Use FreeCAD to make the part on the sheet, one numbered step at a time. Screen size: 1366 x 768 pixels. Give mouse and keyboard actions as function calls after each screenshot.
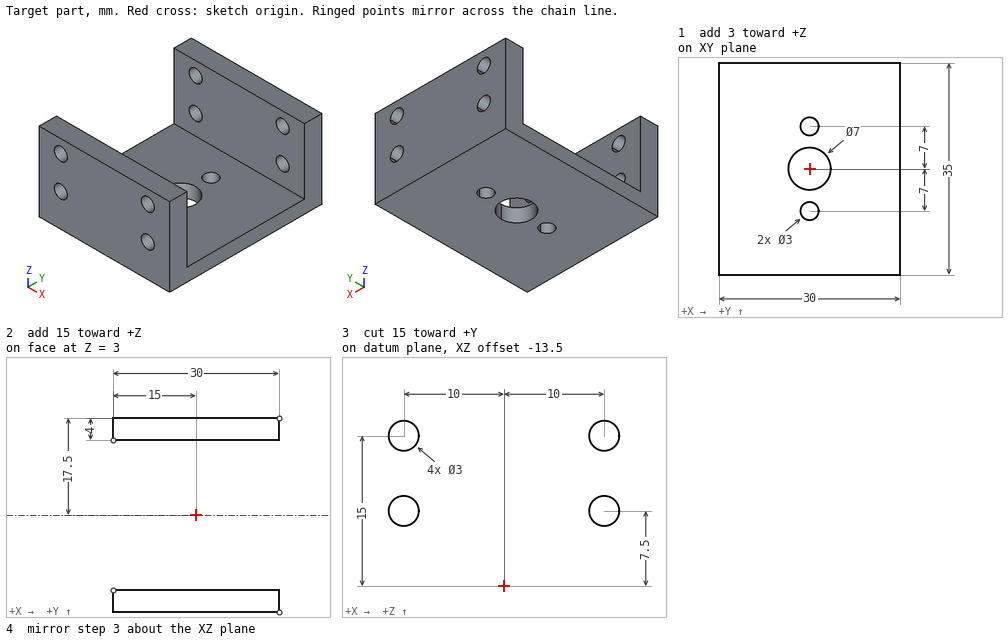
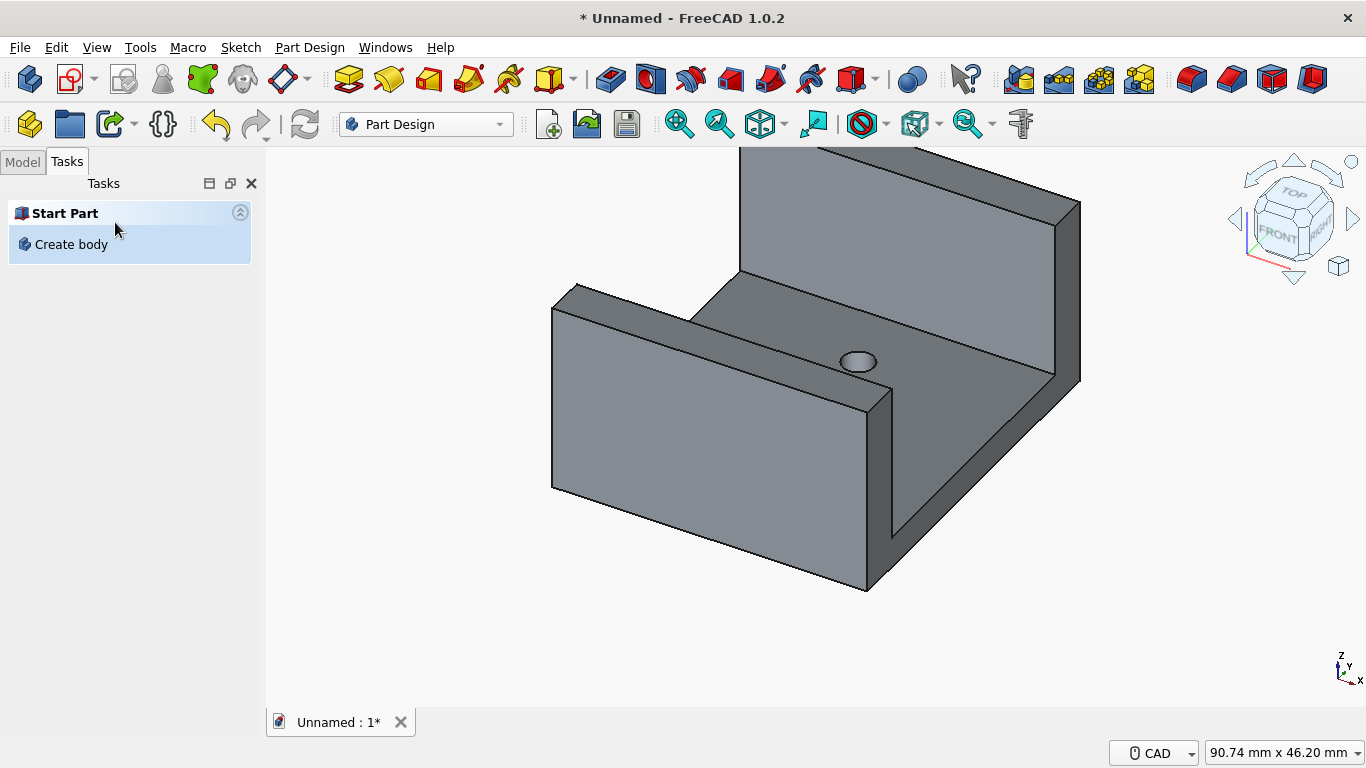
click(680, 124)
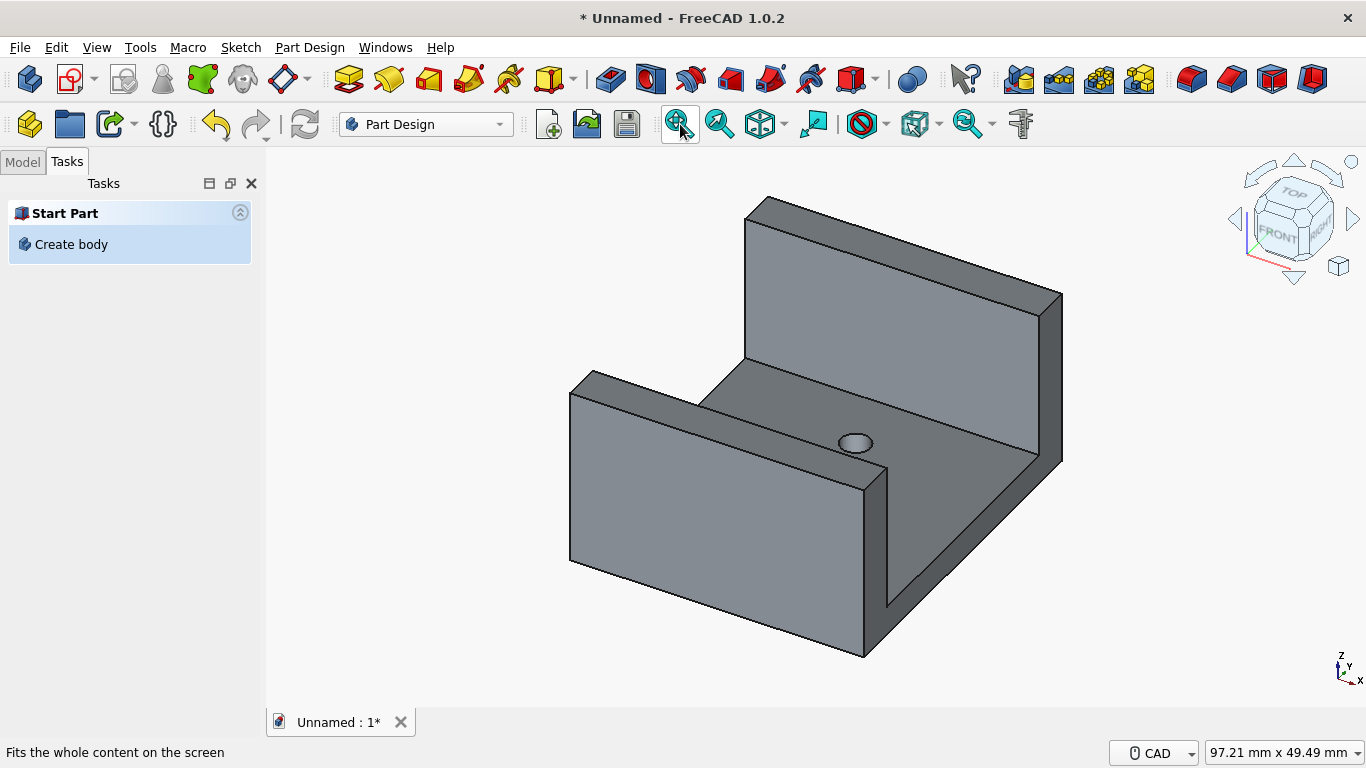
click(23, 161)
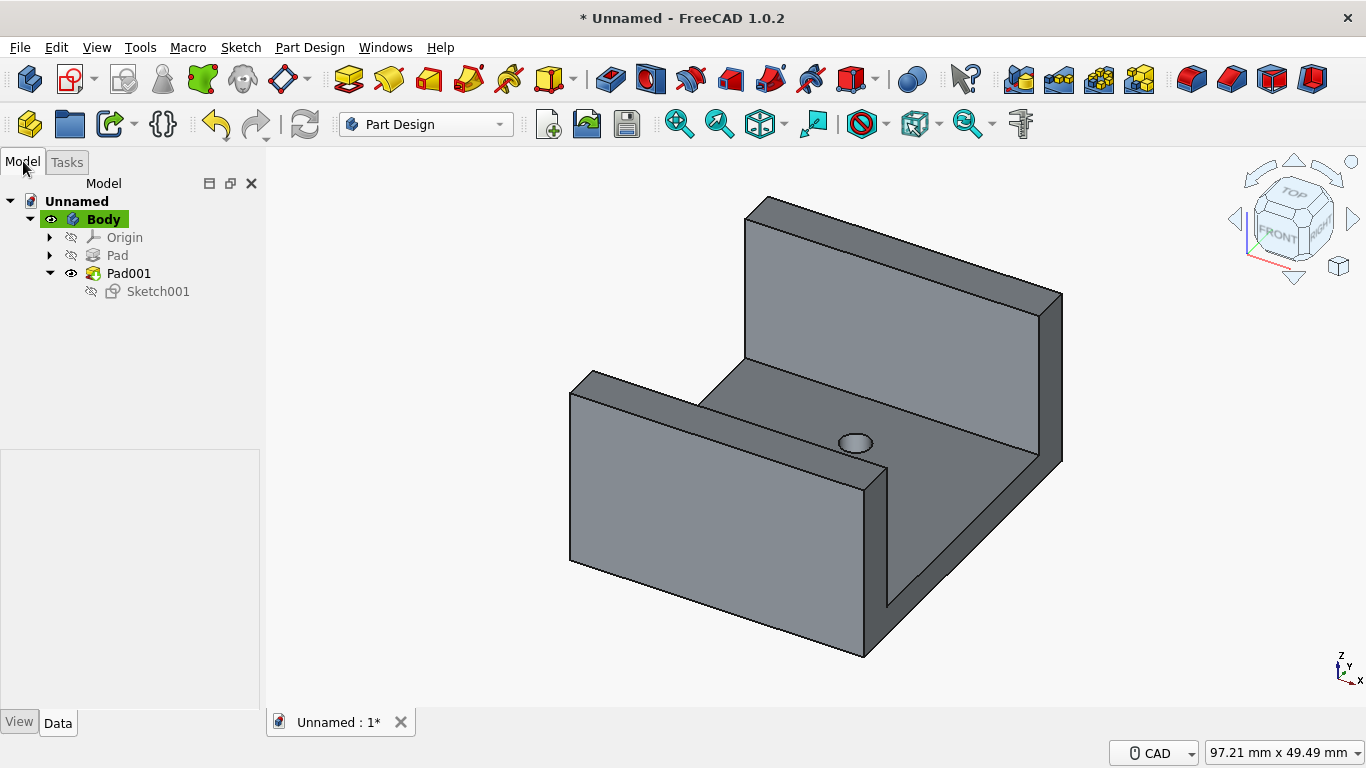
click(50, 237)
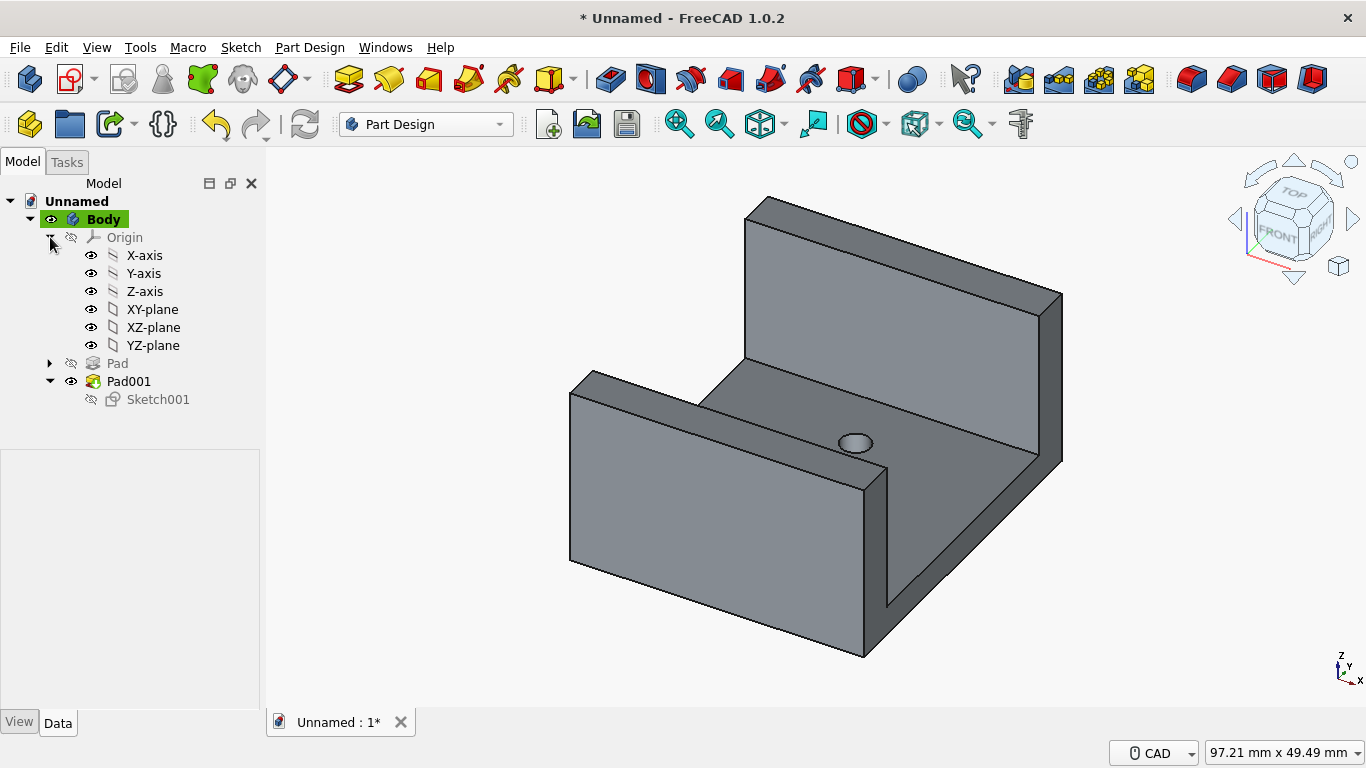
click(136, 327)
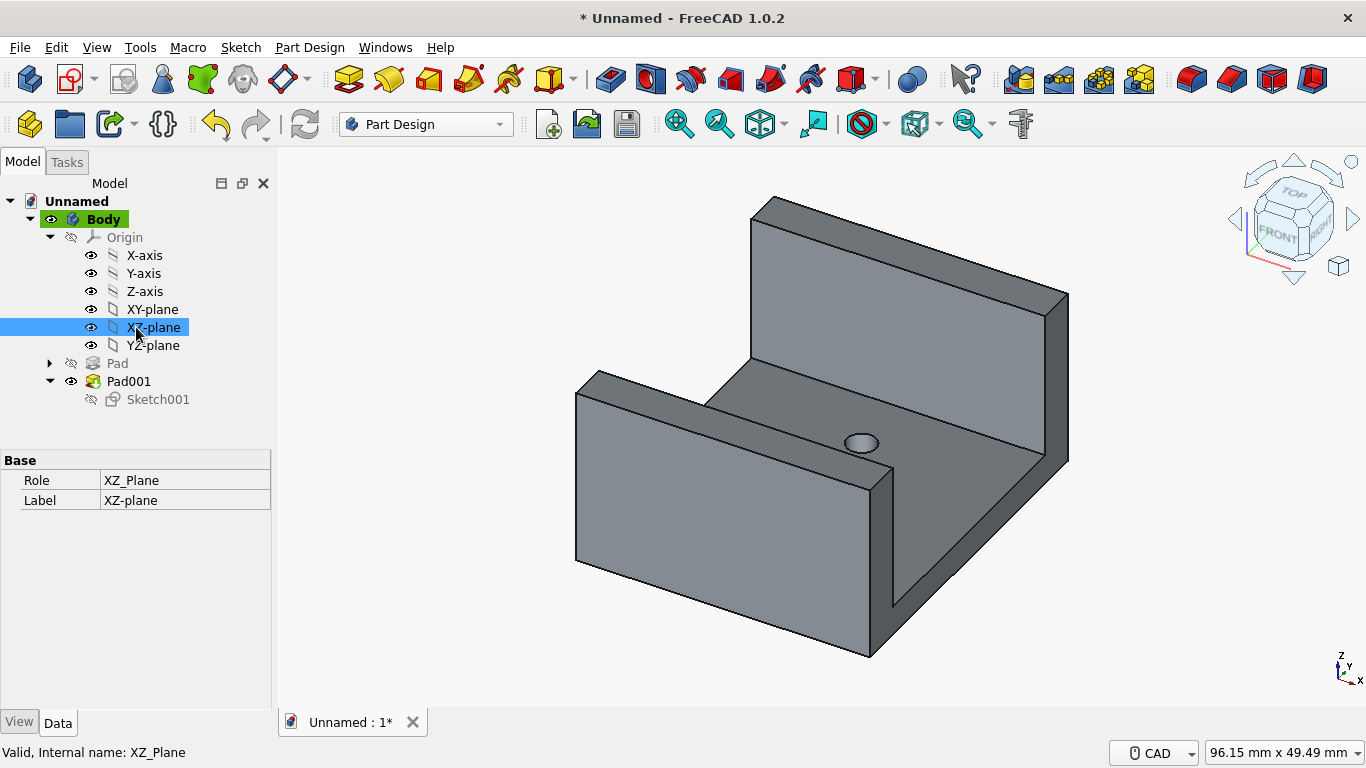
click(284, 80)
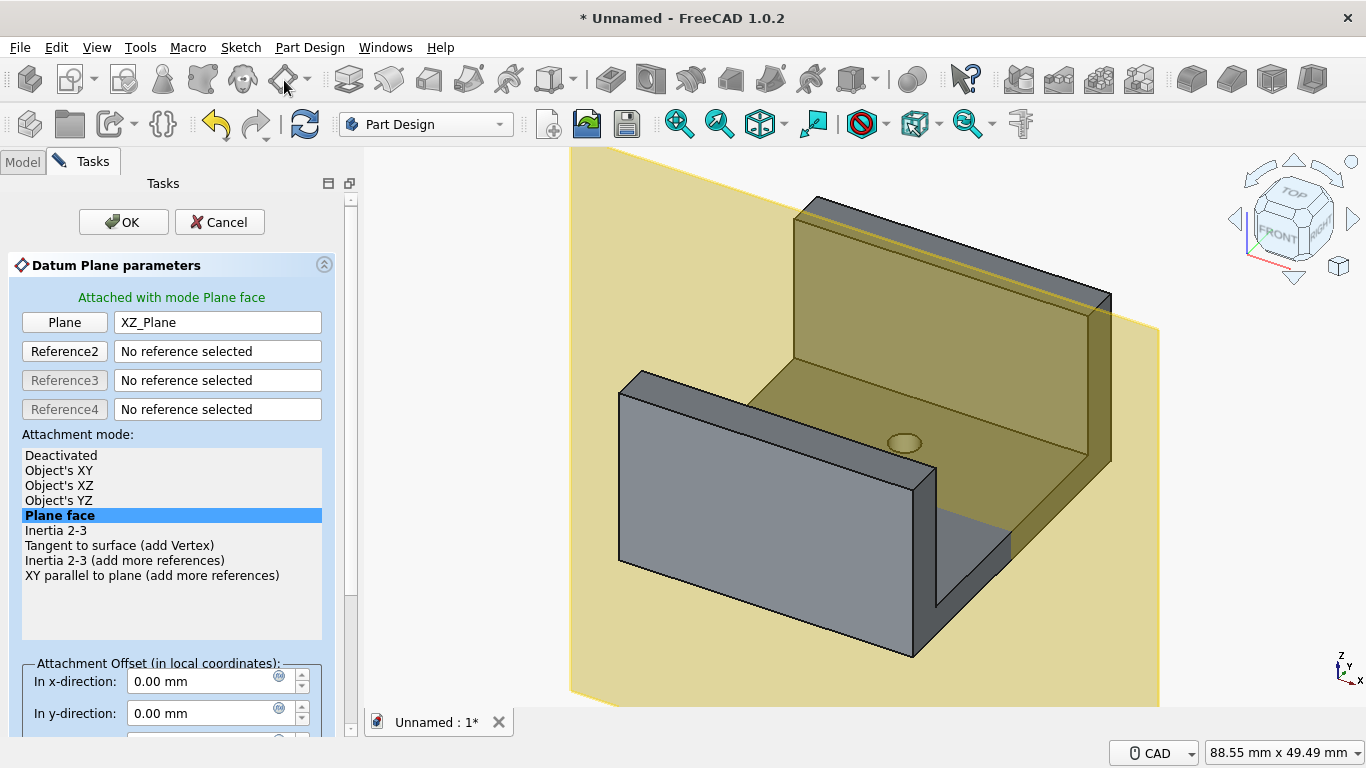
scroll(351, 464, down, 2)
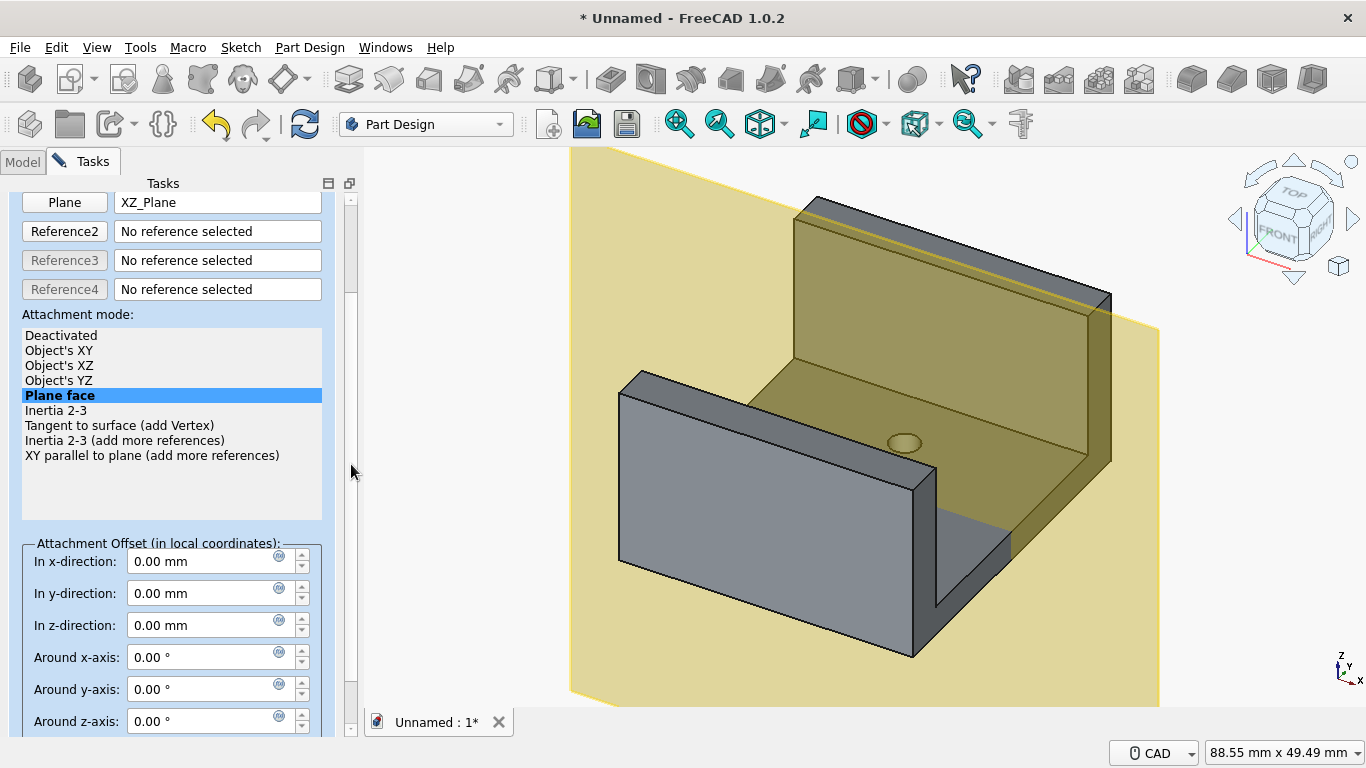
triple_click(210, 625)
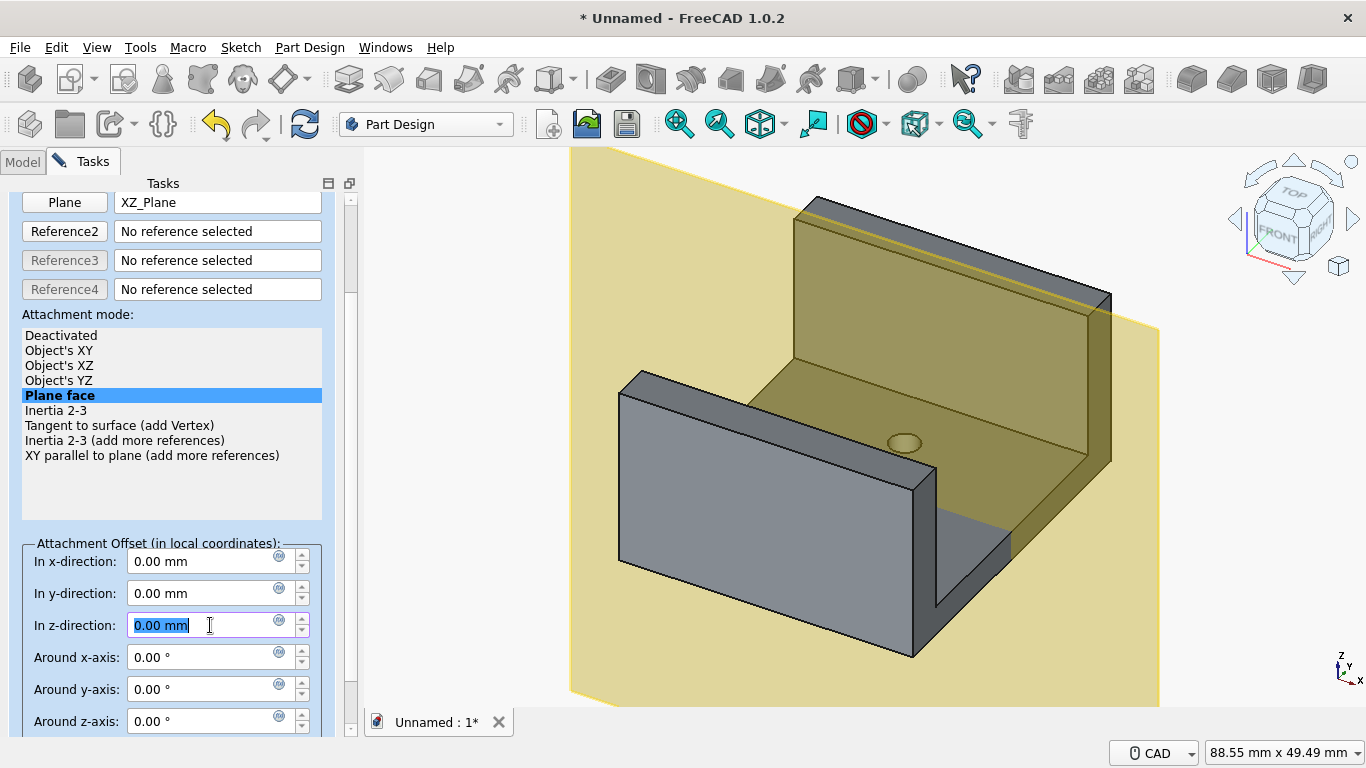
text(-13.5)
key(Tab)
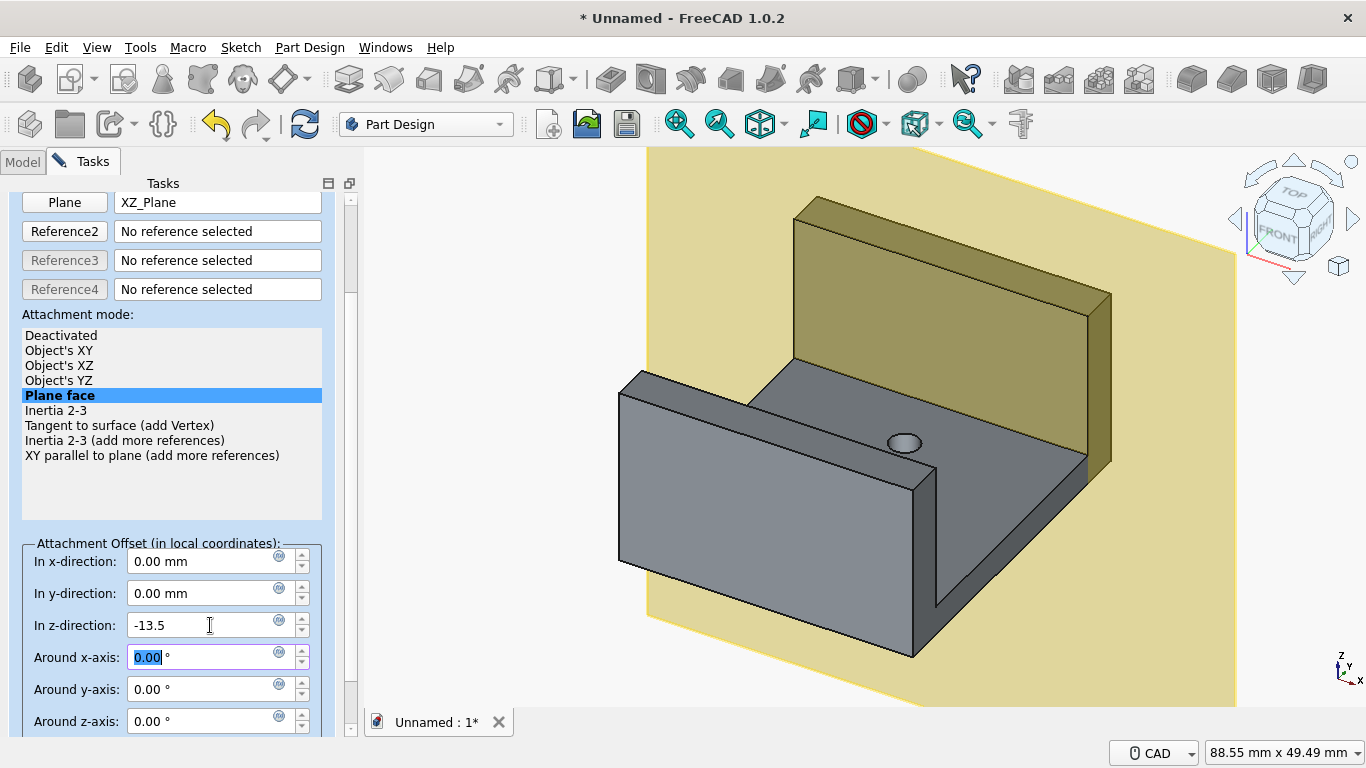
scroll(351, 464, up, 3)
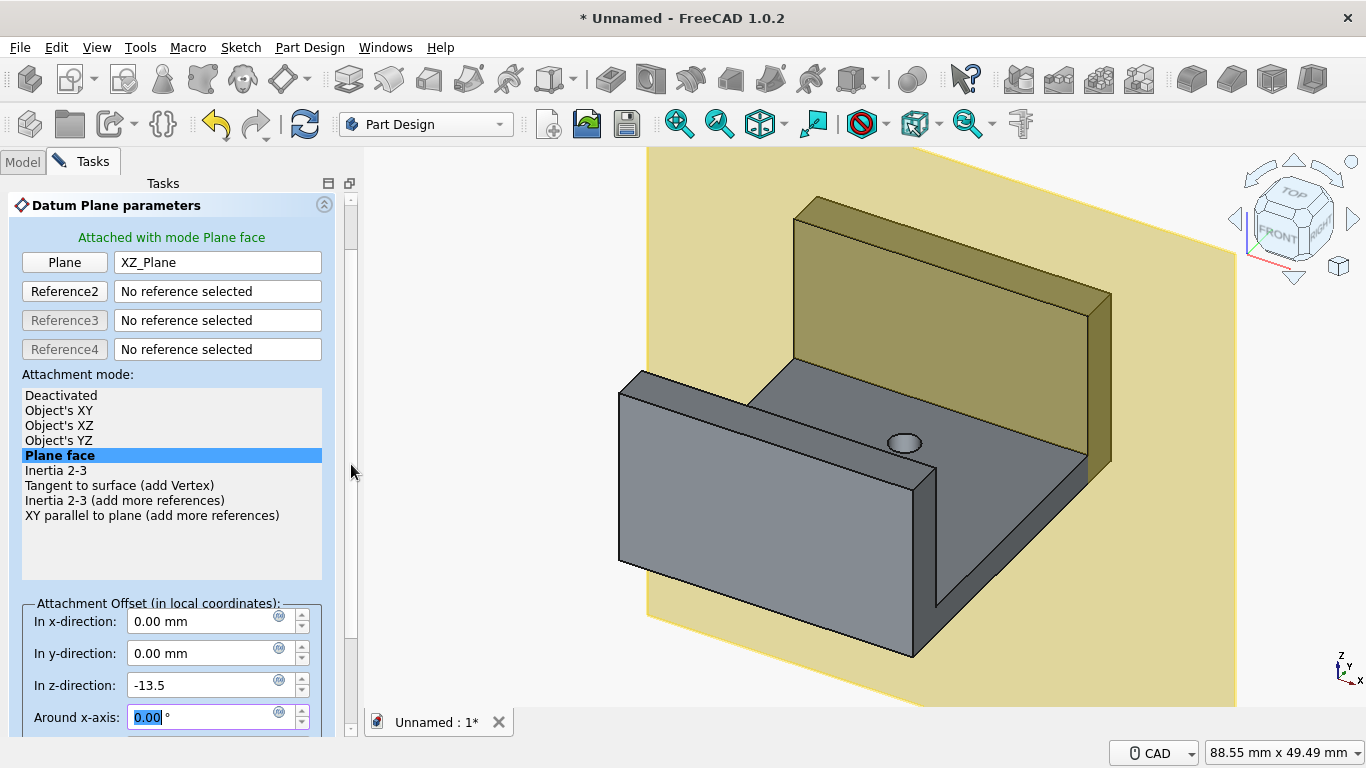
click(124, 222)